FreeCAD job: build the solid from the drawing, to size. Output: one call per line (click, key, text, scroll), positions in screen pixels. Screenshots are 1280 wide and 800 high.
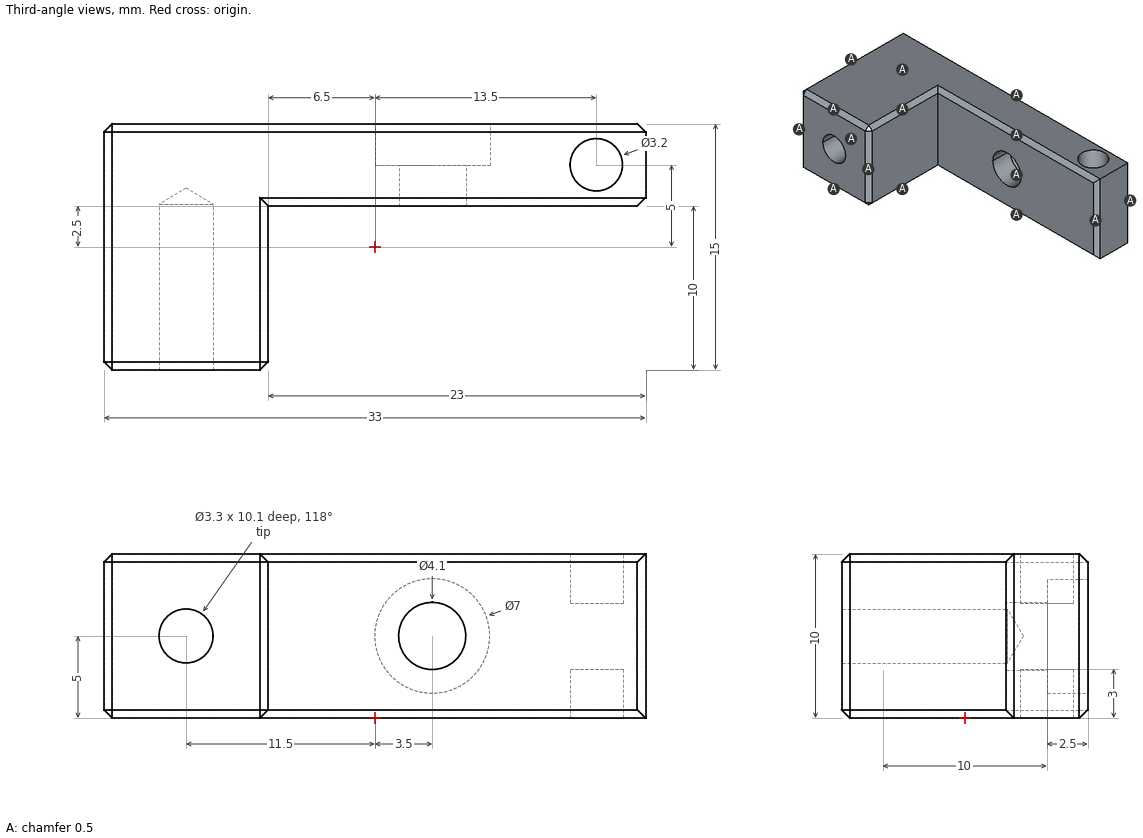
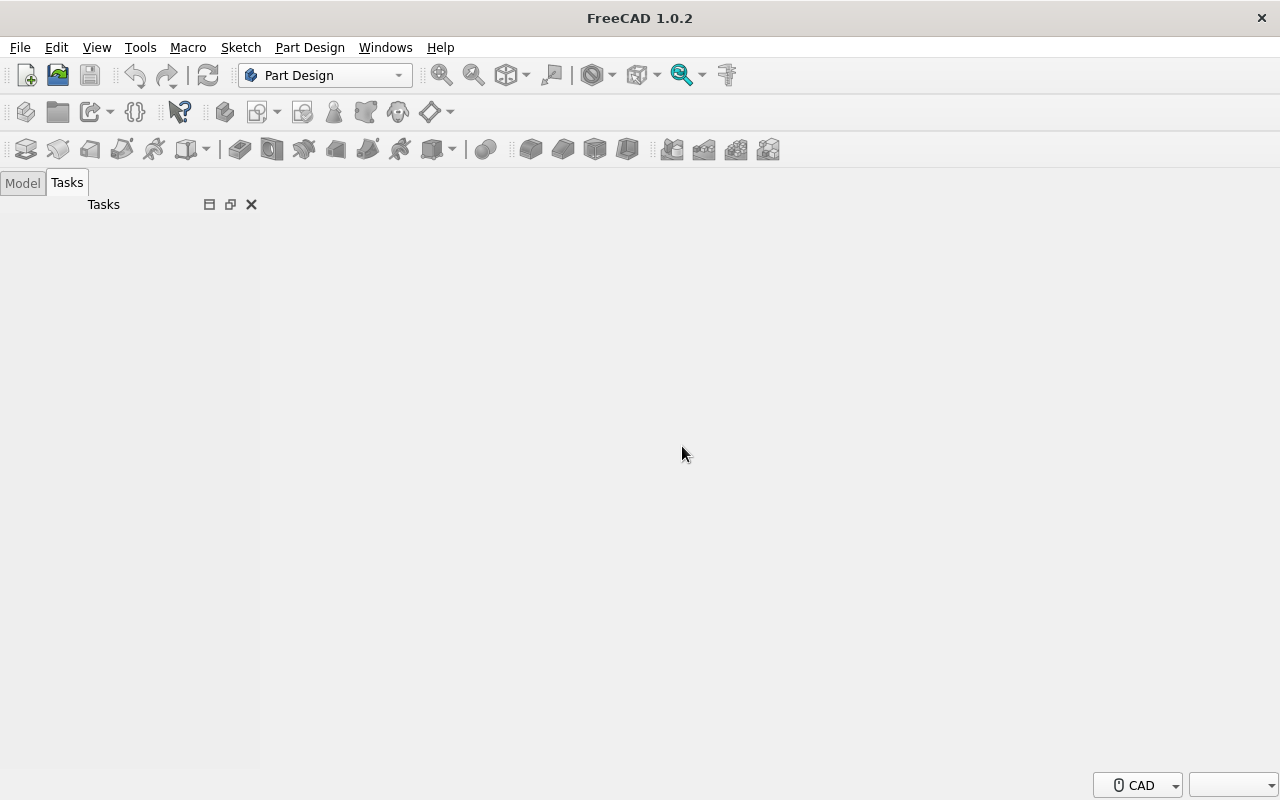
click(26, 76)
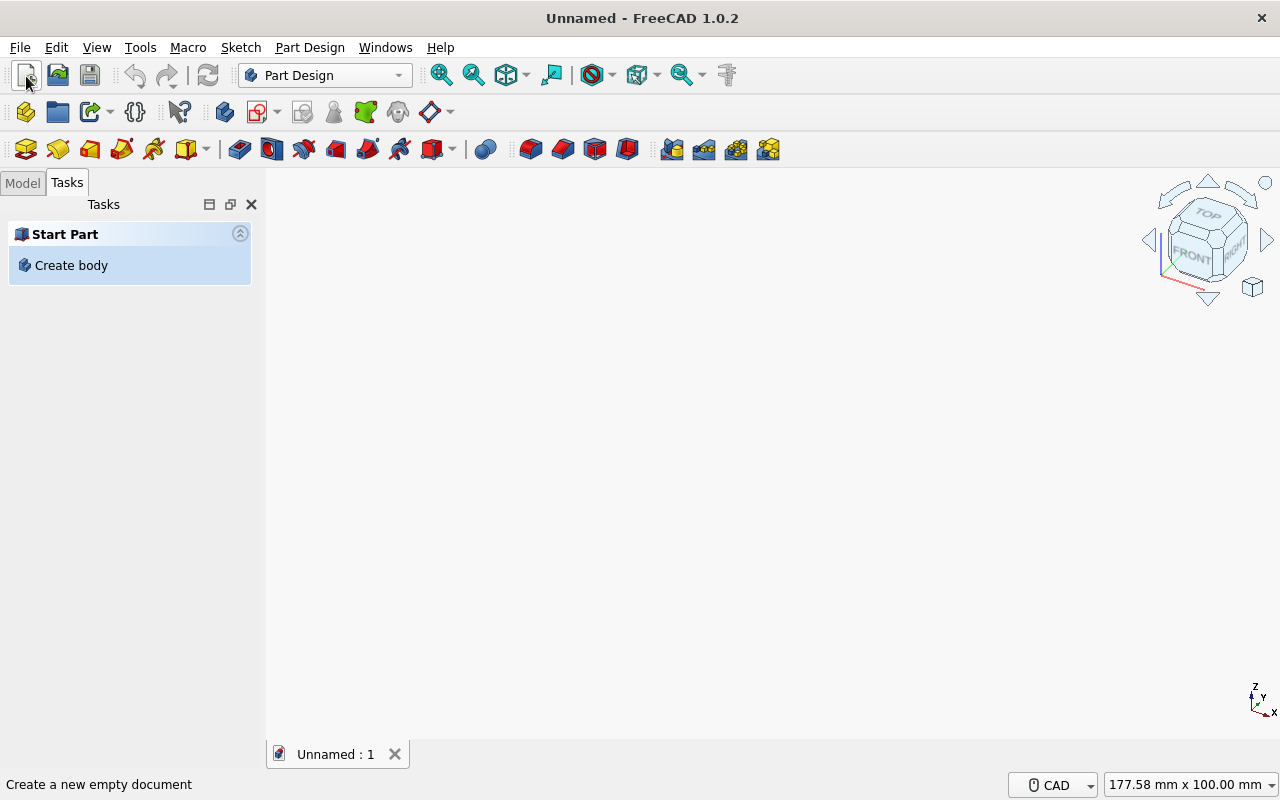
click(258, 112)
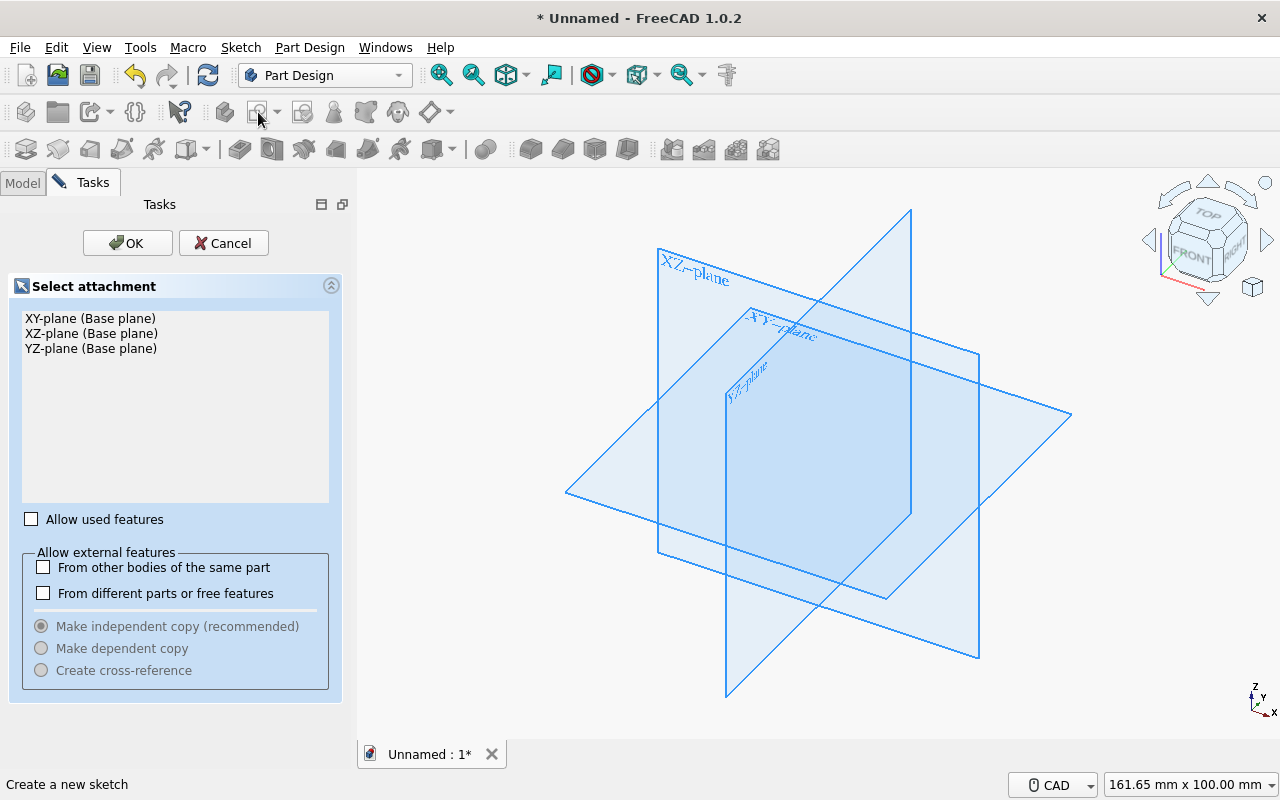
click(82, 318)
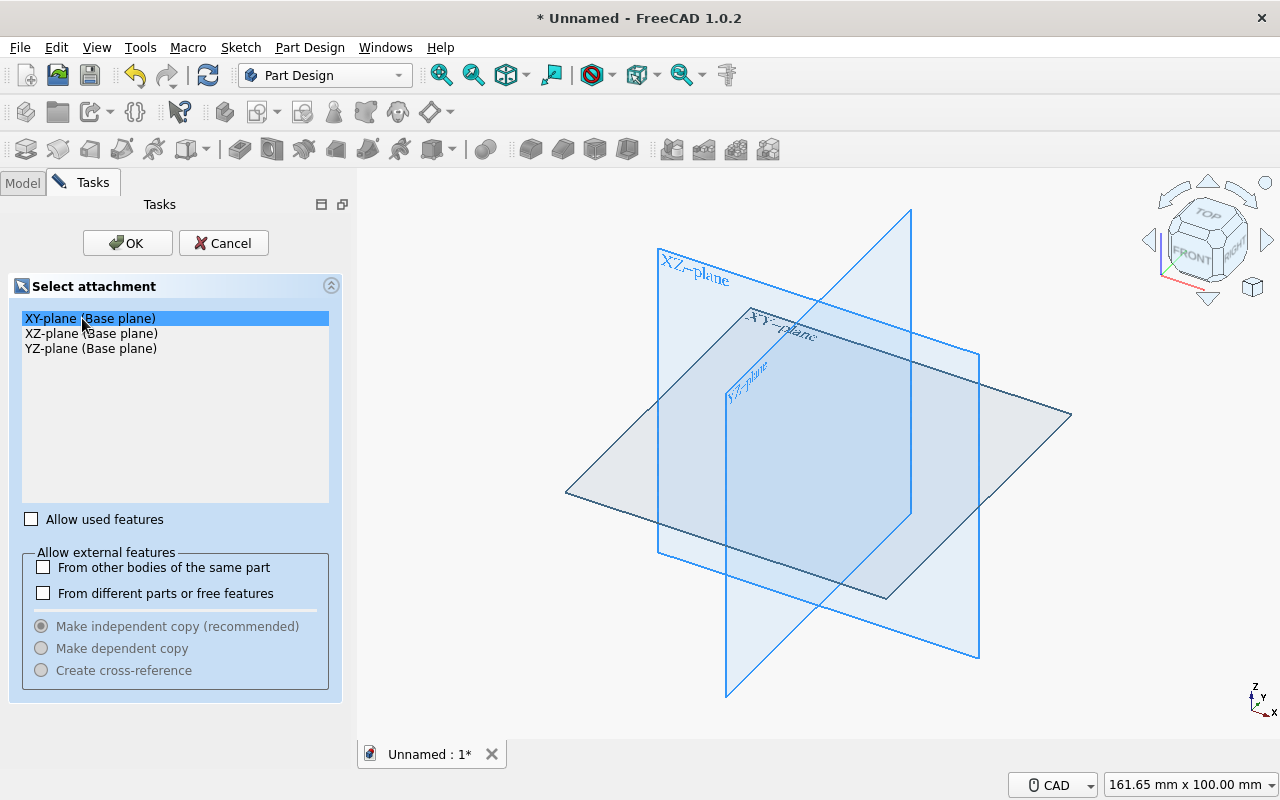
click(128, 243)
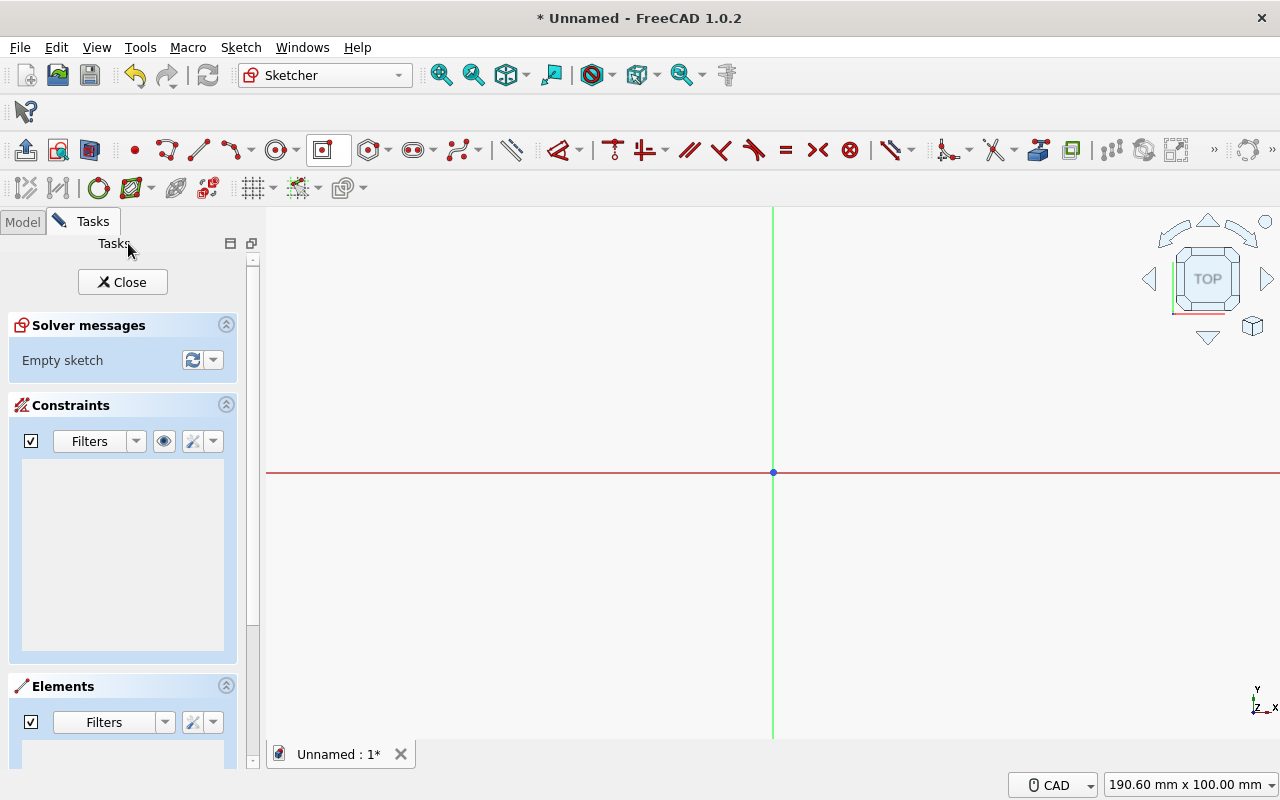
scroll(803, 473, up, 6)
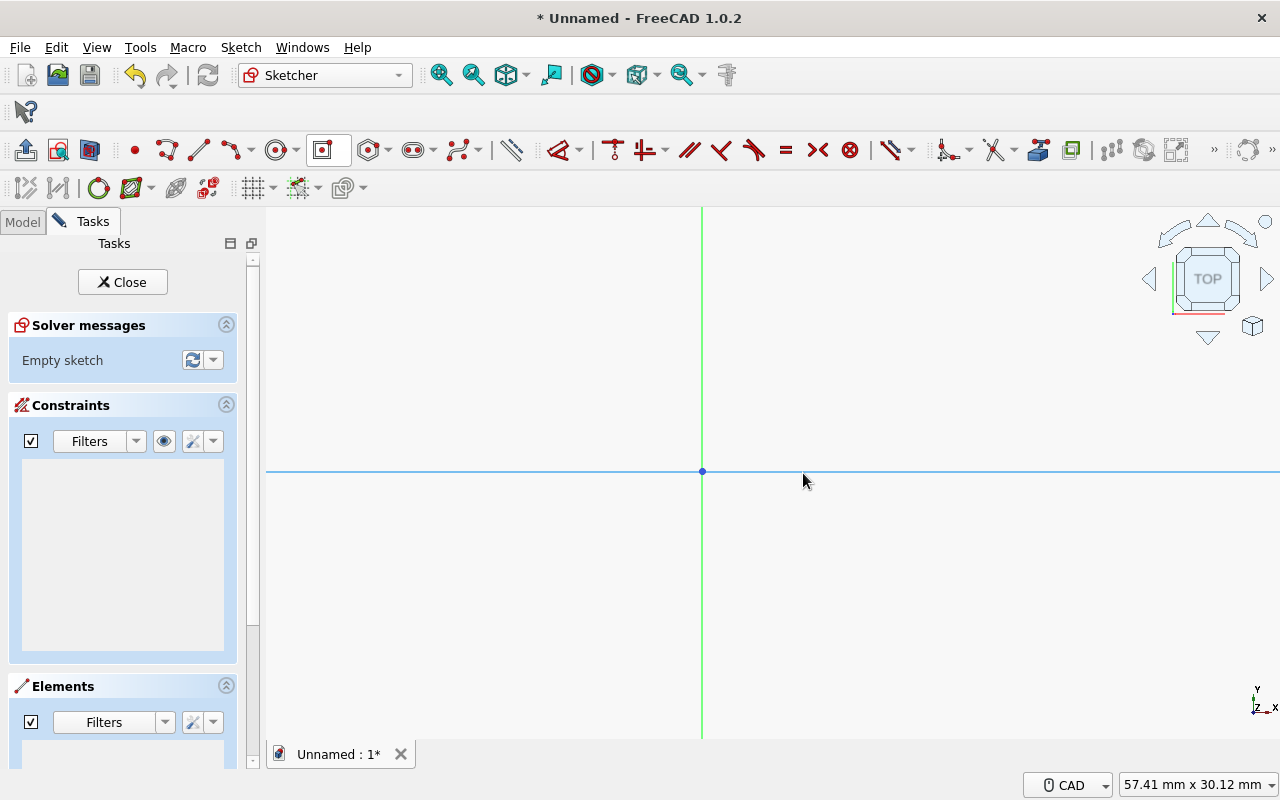
click(322, 150)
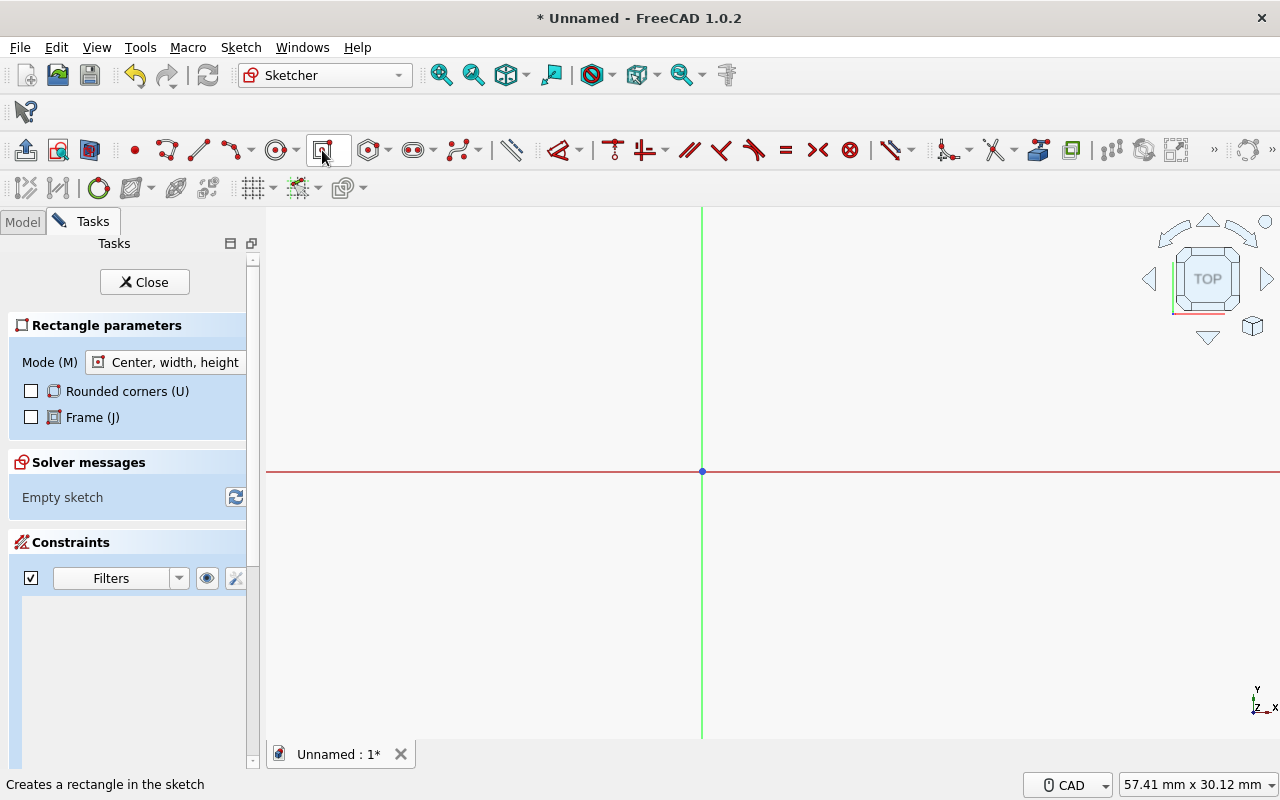
click(702, 472)
move(994, 339)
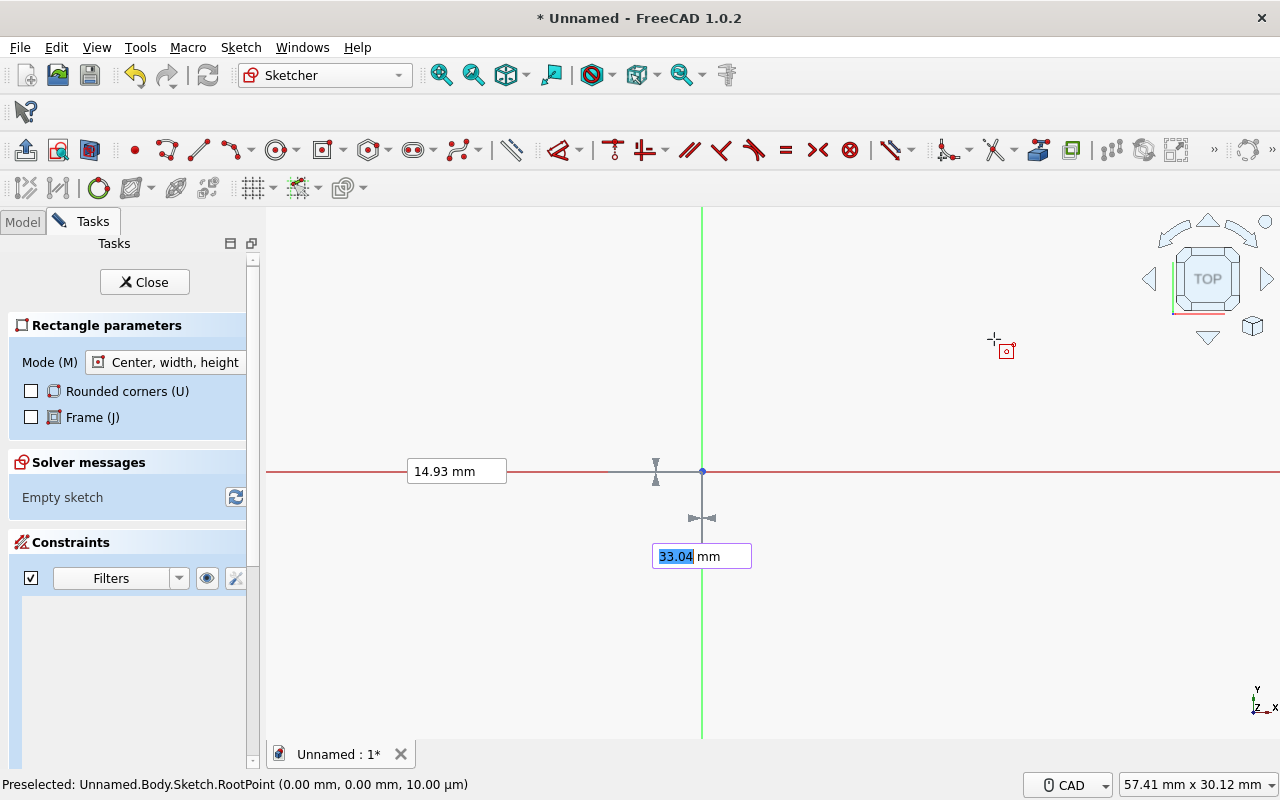
text(33)
key(Tab)
text(15)
key(Return)
key(Escape)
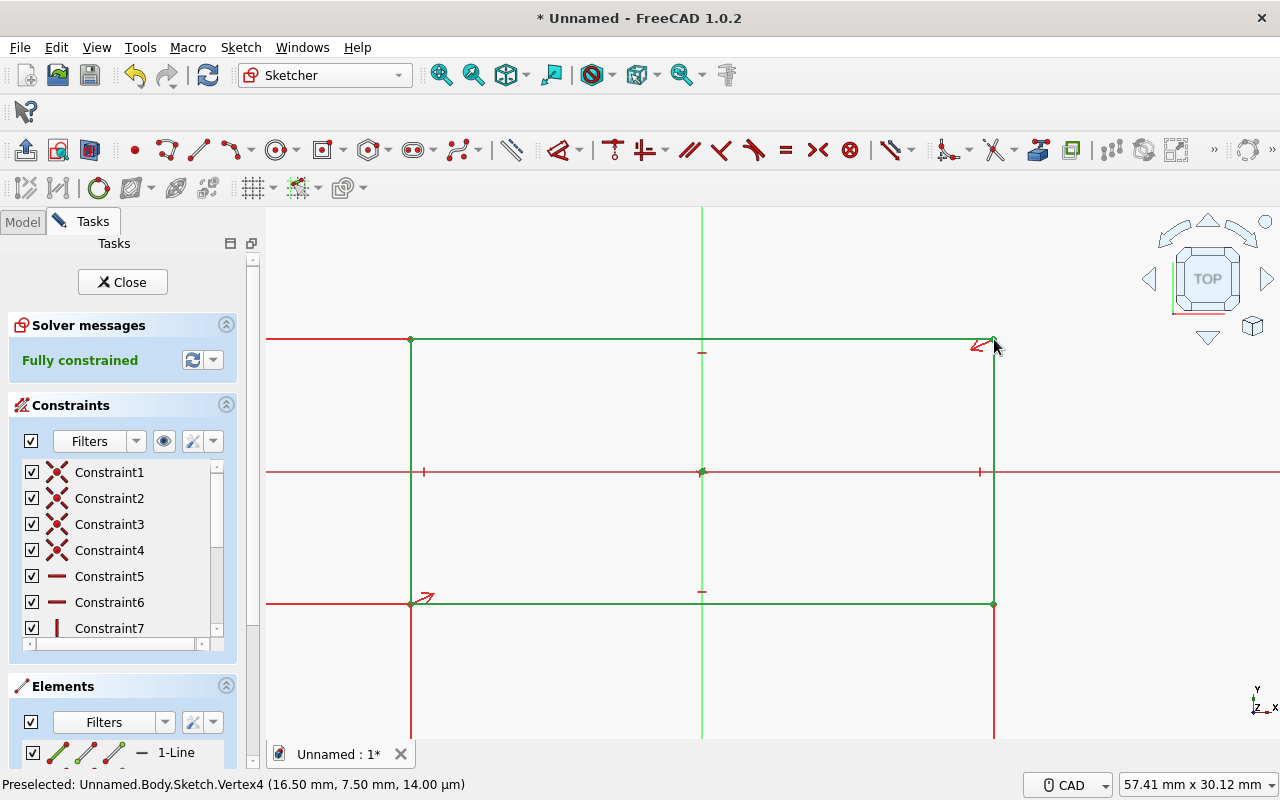
click(123, 282)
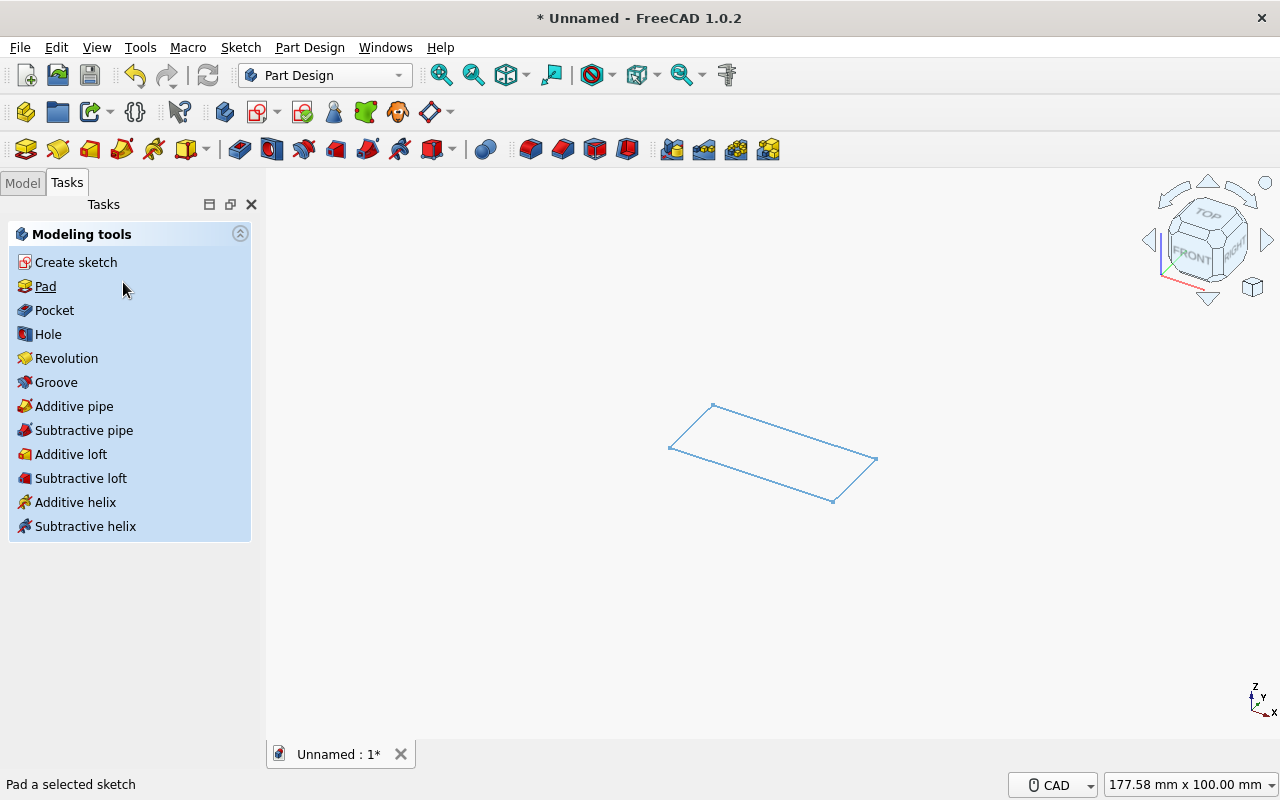
click(26, 150)